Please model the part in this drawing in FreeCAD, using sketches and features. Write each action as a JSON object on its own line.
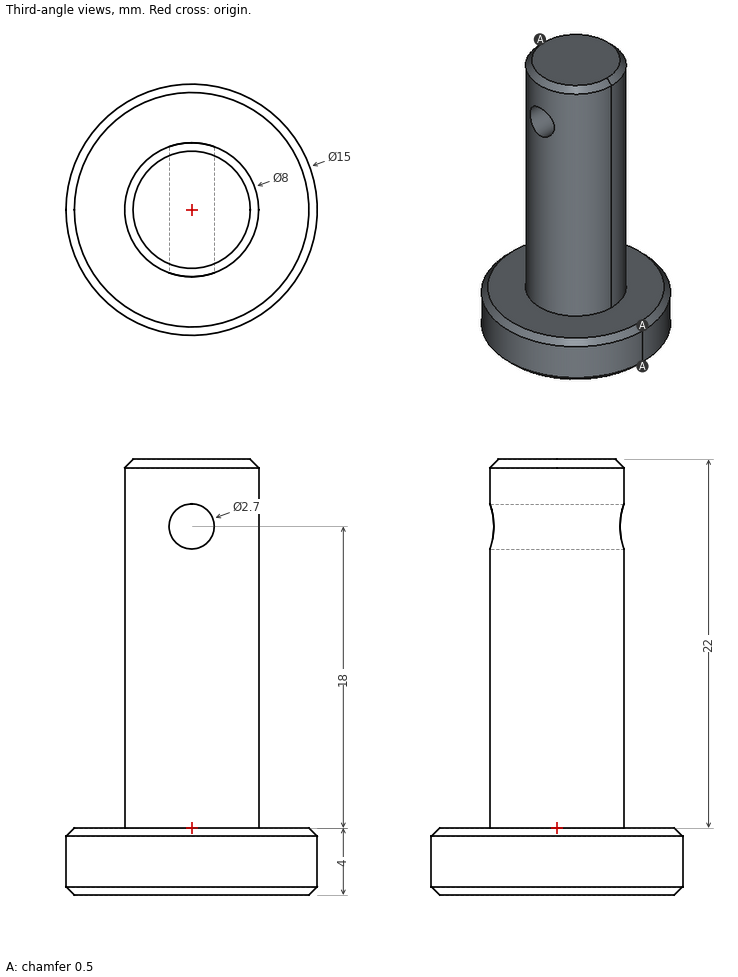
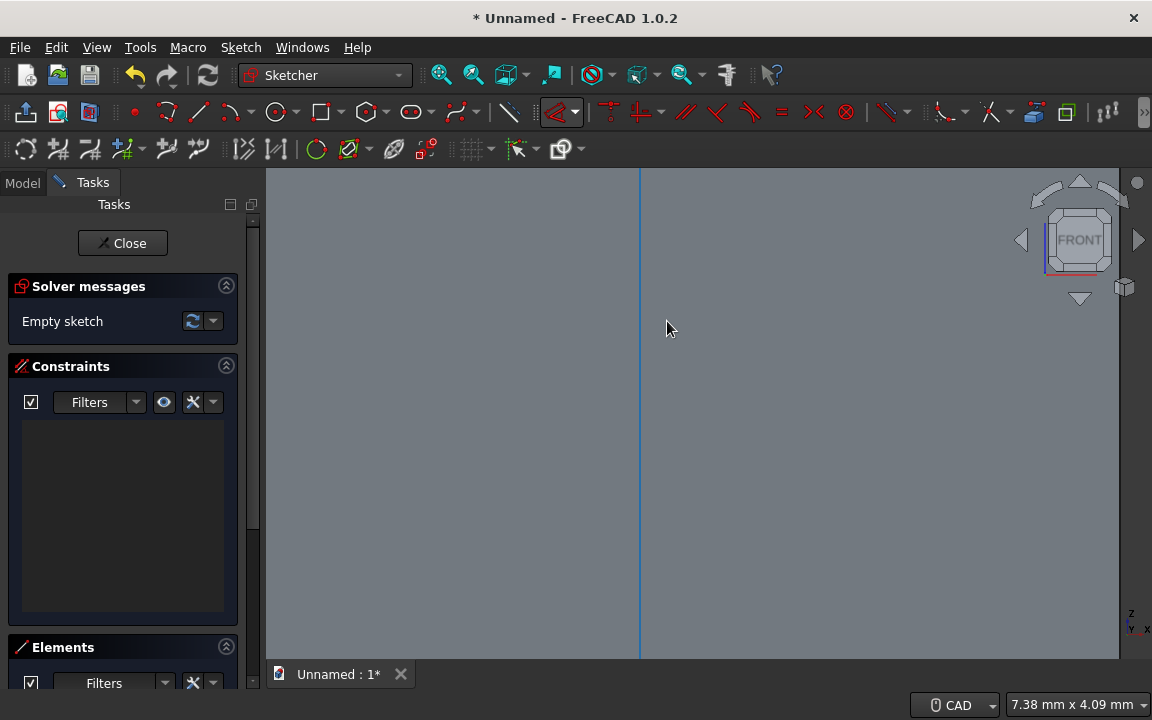
{"action": "left_click", "coordinate": [276, 112]}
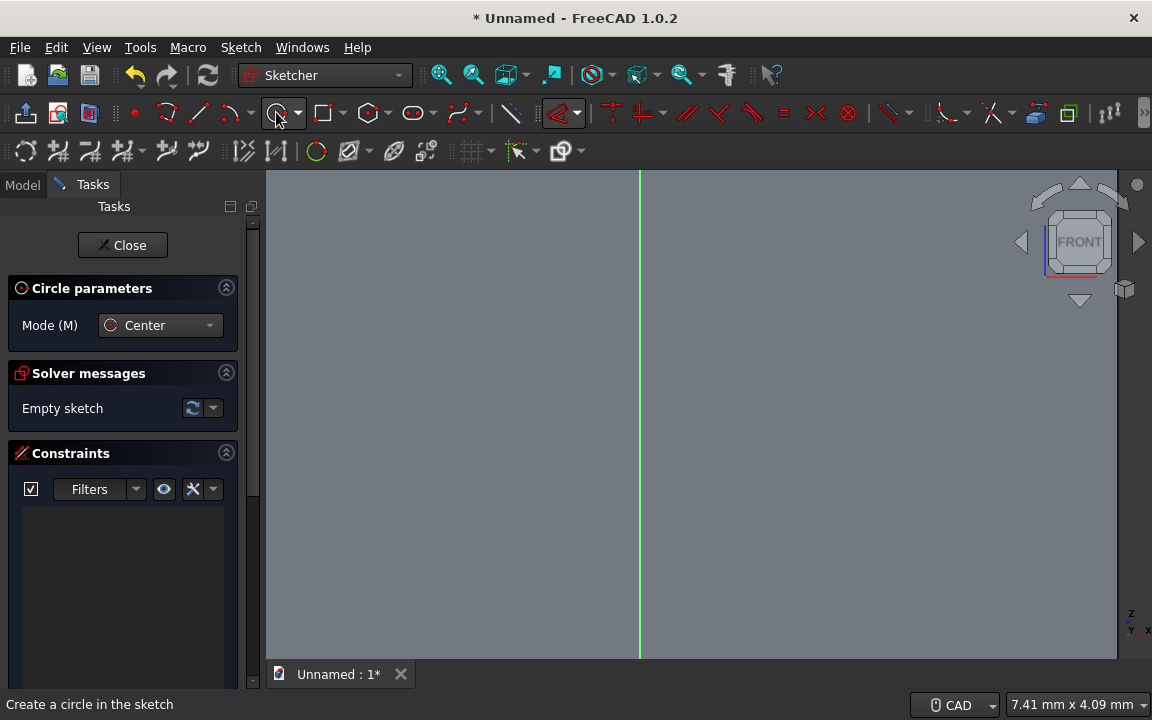
{"action": "left_click", "coordinate": [640, 408]}
{"action": "left_click", "coordinate": [754, 294]}
{"action": "key", "text": "Escape"}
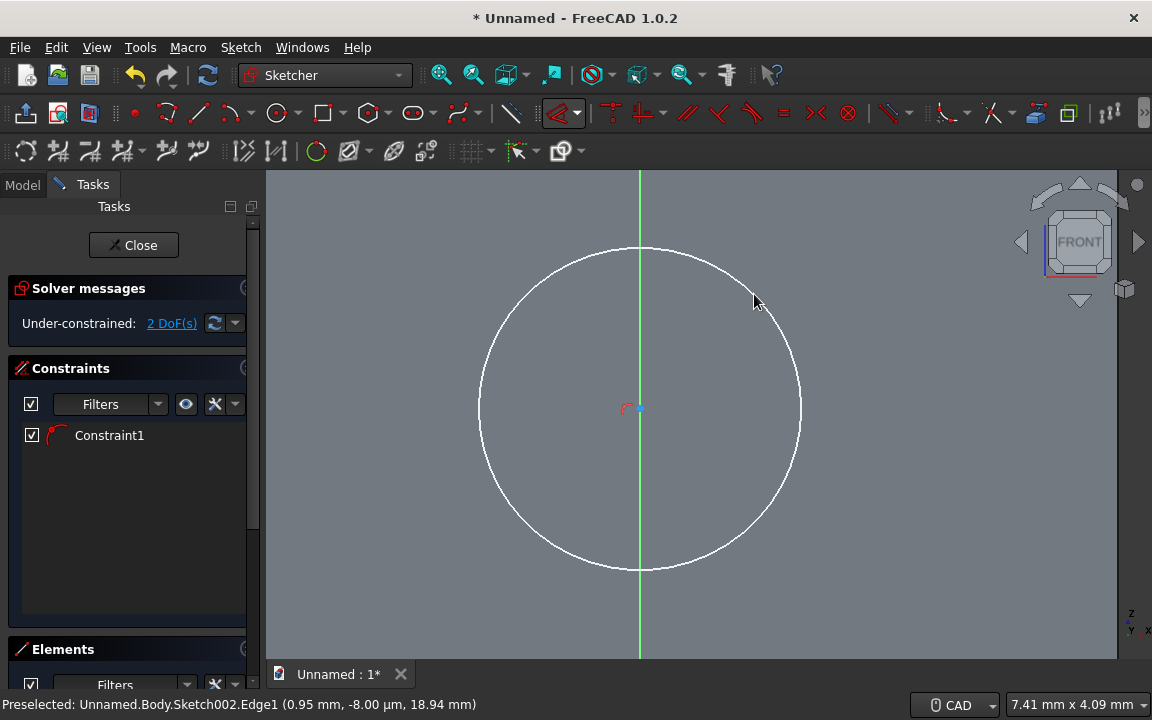
{"action": "left_click", "coordinate": [754, 295]}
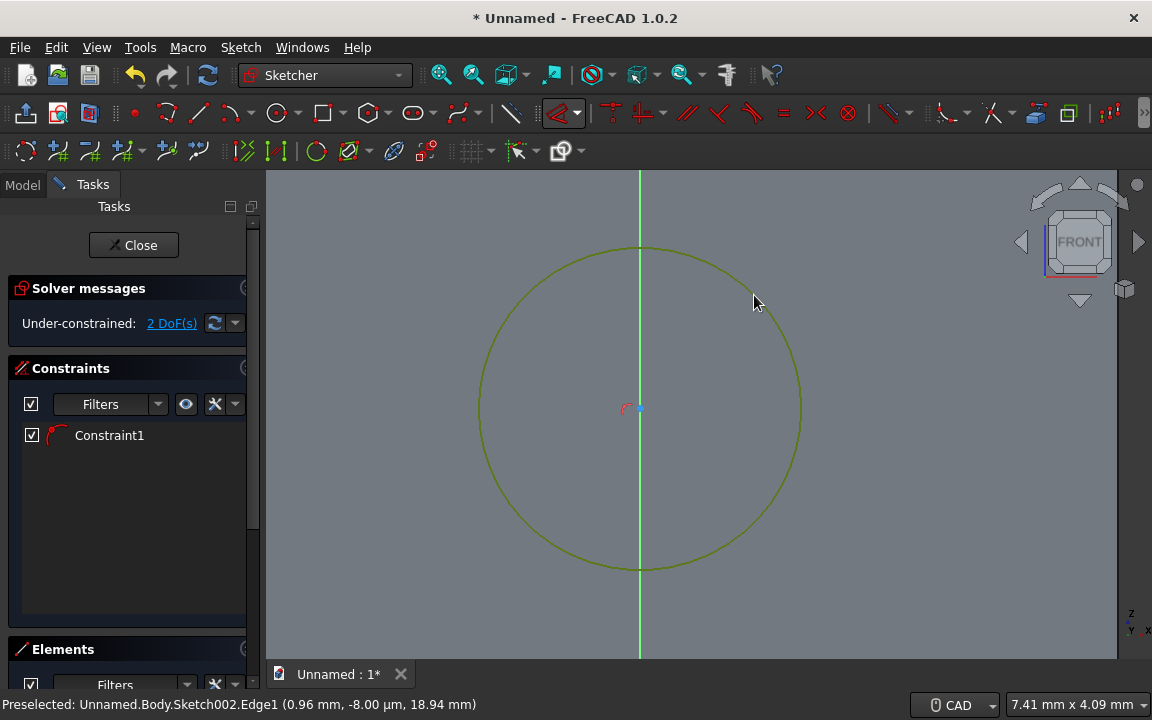
{"action": "left_click", "coordinate": [580, 114]}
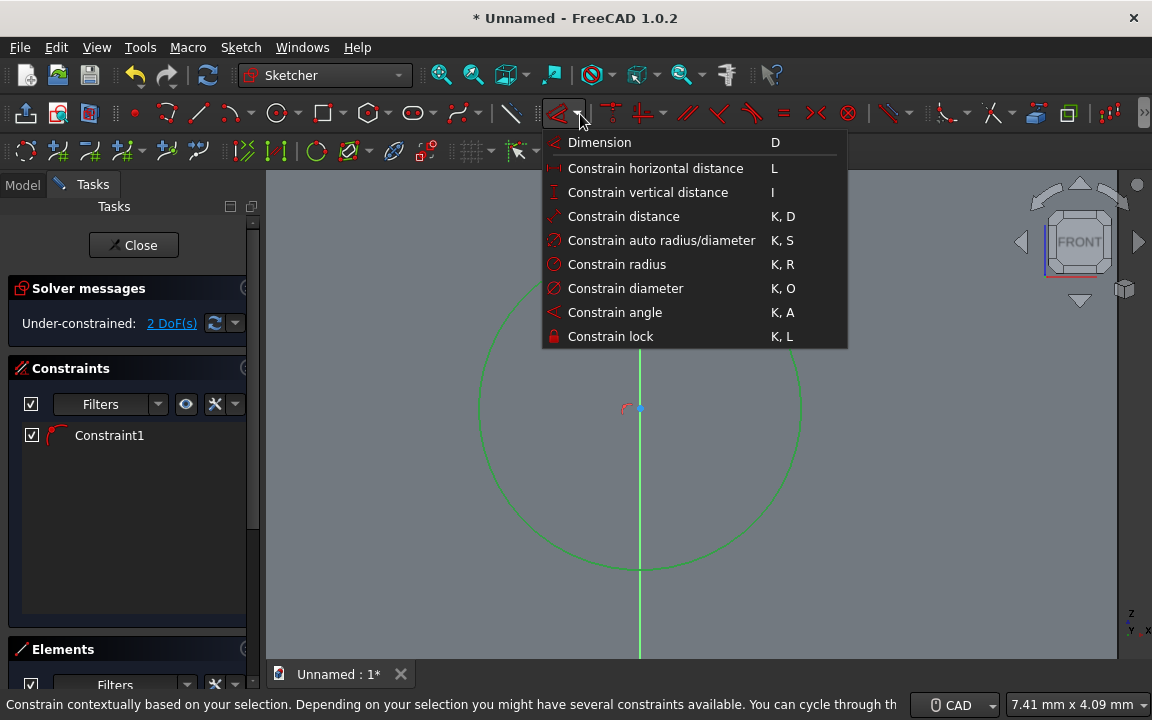
{"action": "left_click", "coordinate": [695, 288]}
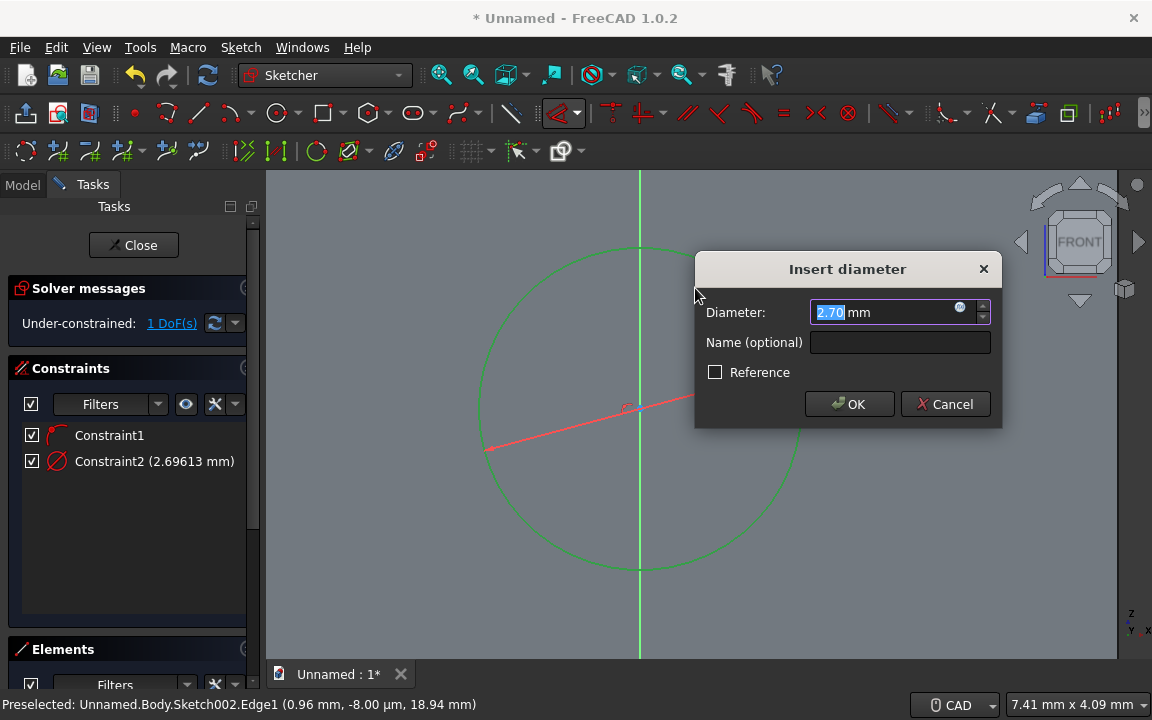
{"action": "type", "text": "2.7"}
{"action": "key", "text": "Return"}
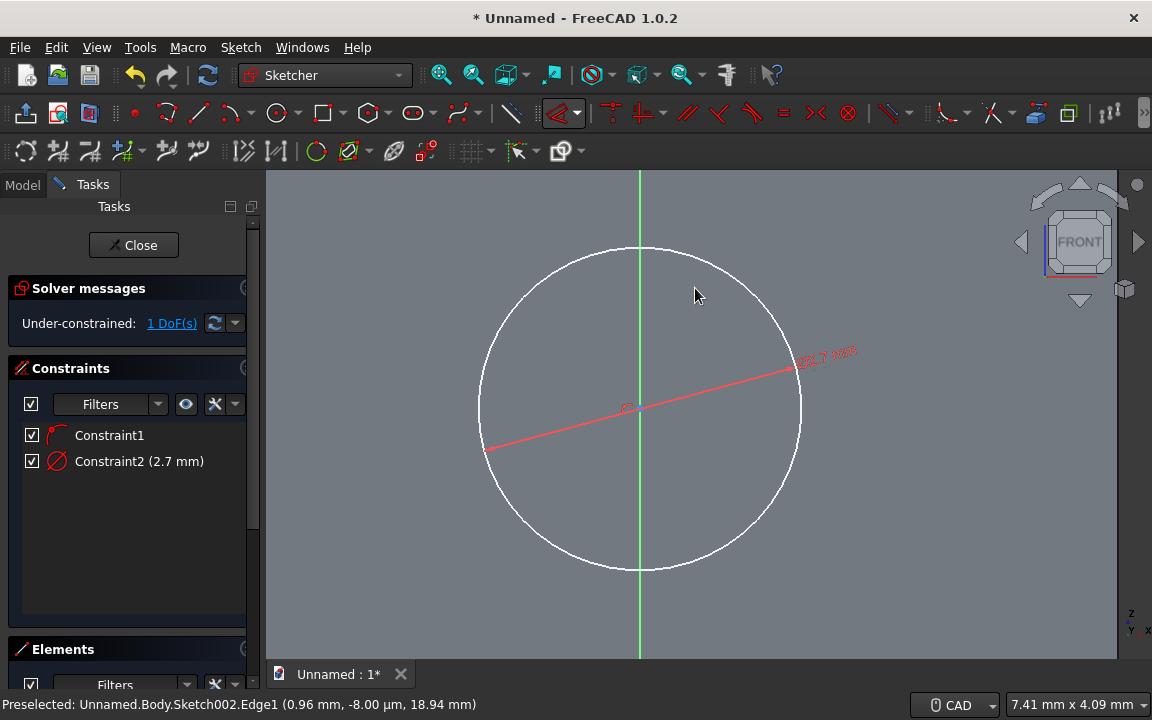
{"action": "left_click", "coordinate": [640, 409]}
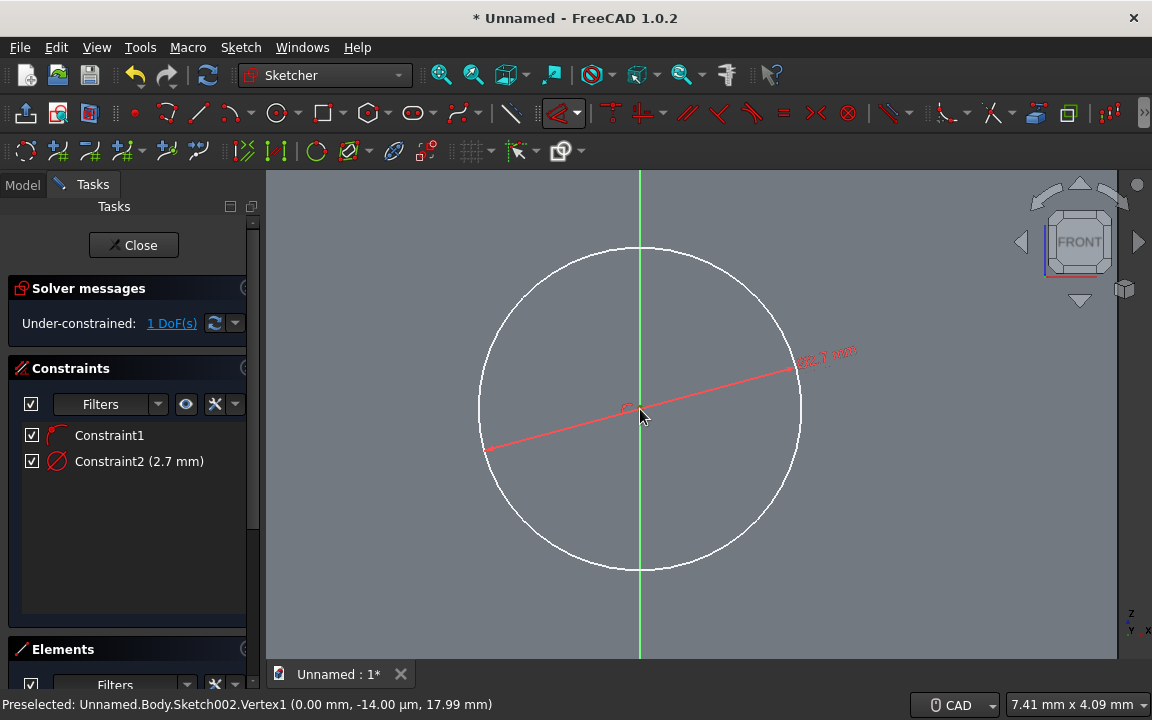
{"action": "left_click", "coordinate": [580, 114]}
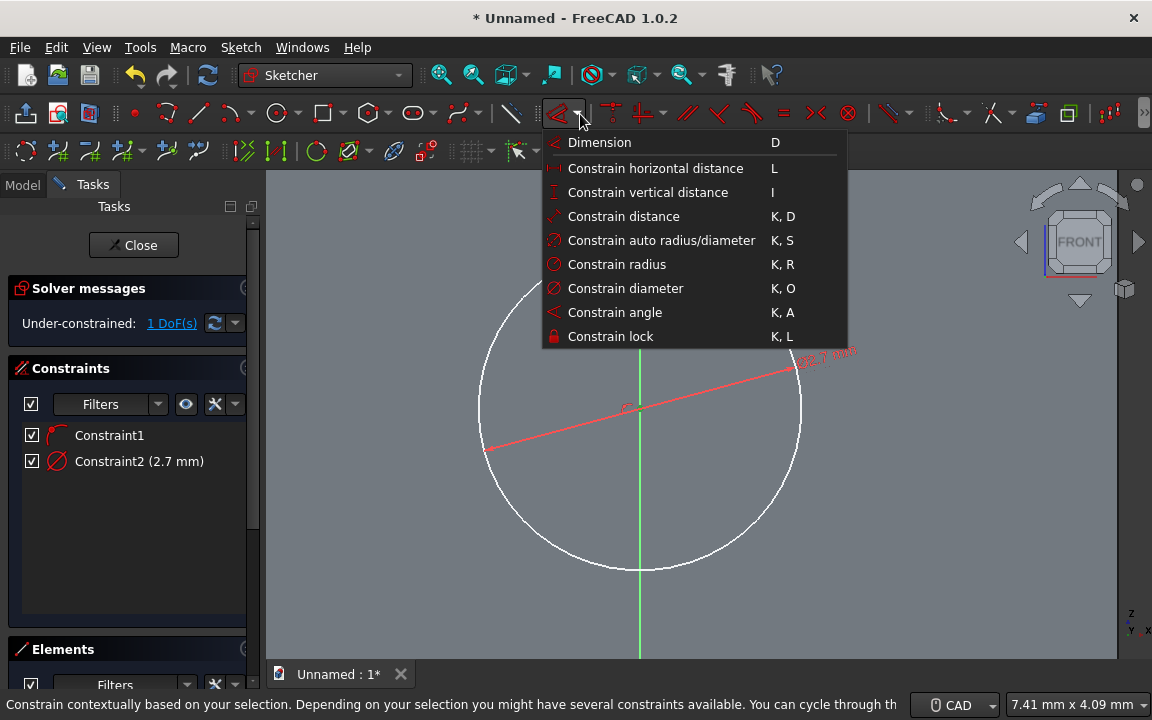
{"action": "left_click", "coordinate": [695, 192]}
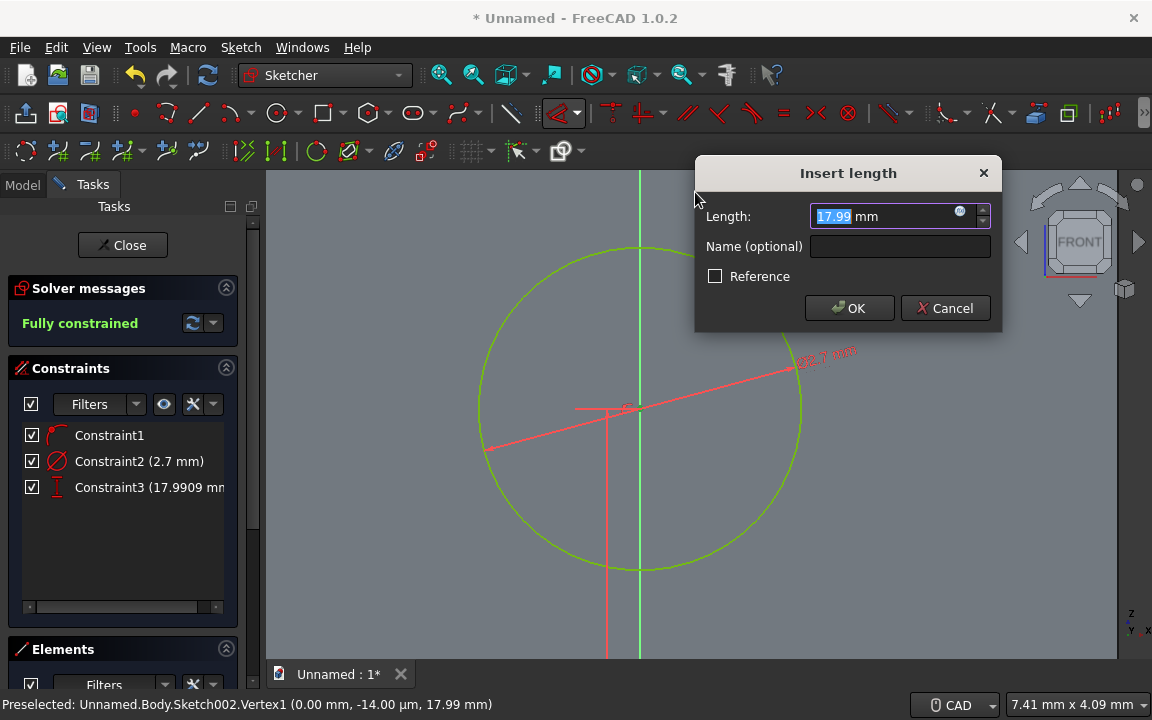
{"action": "type", "text": "18"}
{"action": "key", "text": "Return"}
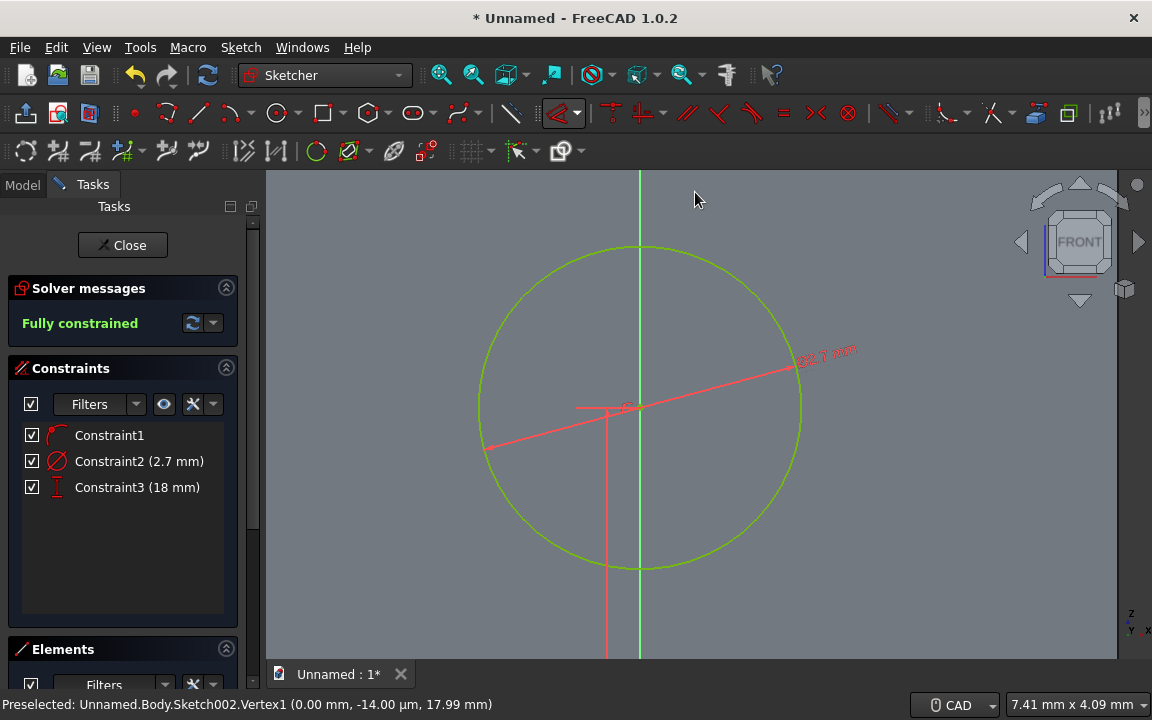
{"action": "left_click", "coordinate": [123, 245]}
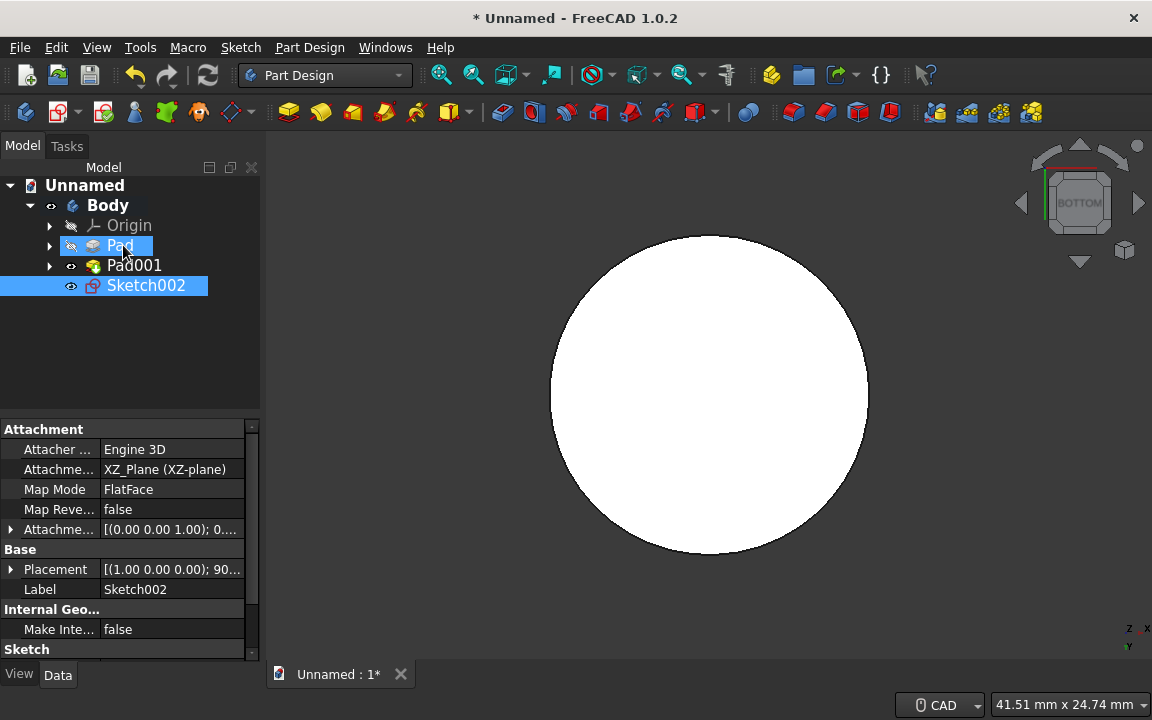
{"action": "left_click", "coordinate": [504, 112]}